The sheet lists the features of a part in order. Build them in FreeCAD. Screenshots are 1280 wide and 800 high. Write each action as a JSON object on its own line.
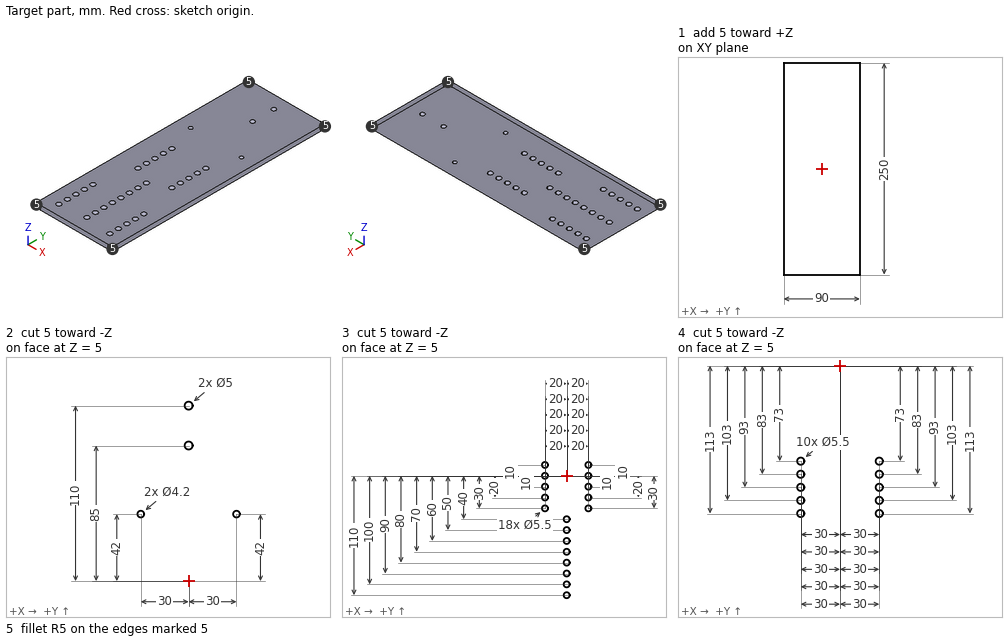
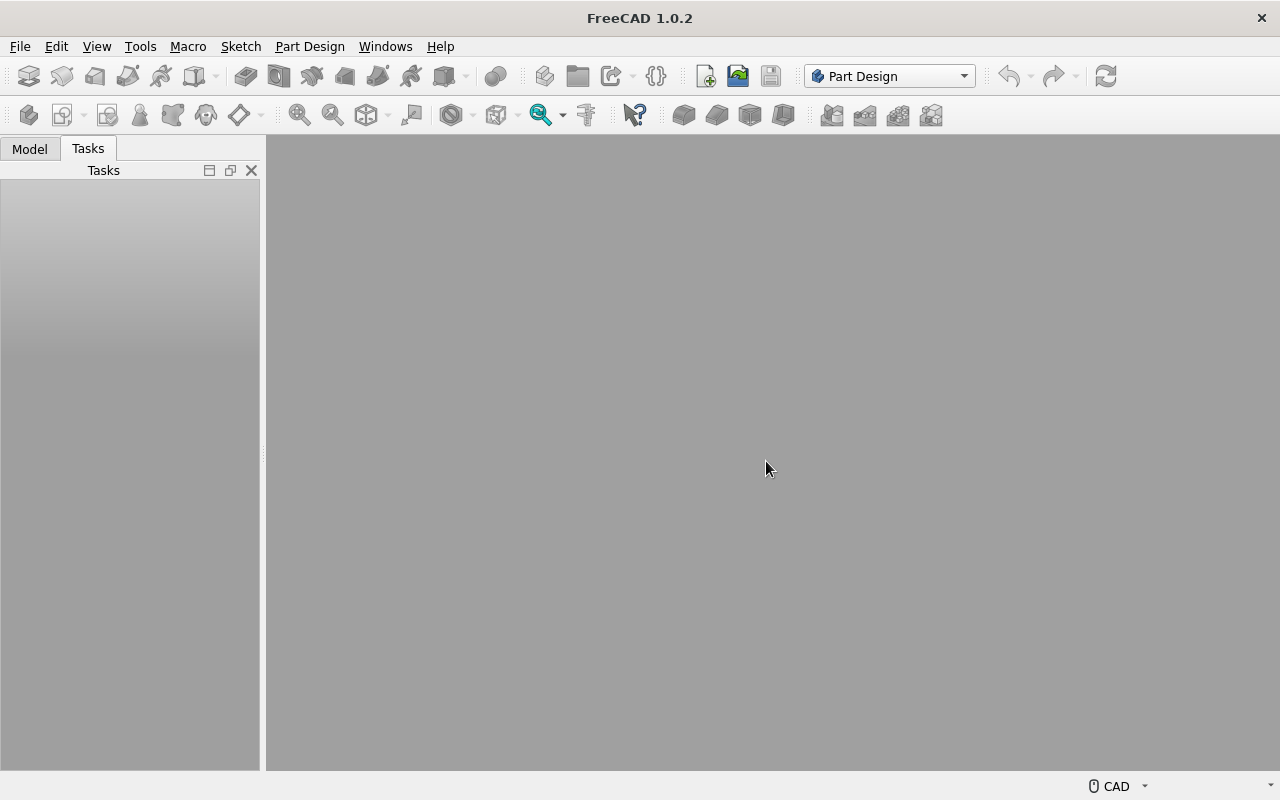
{"action": "key", "text": "ctrl+n"}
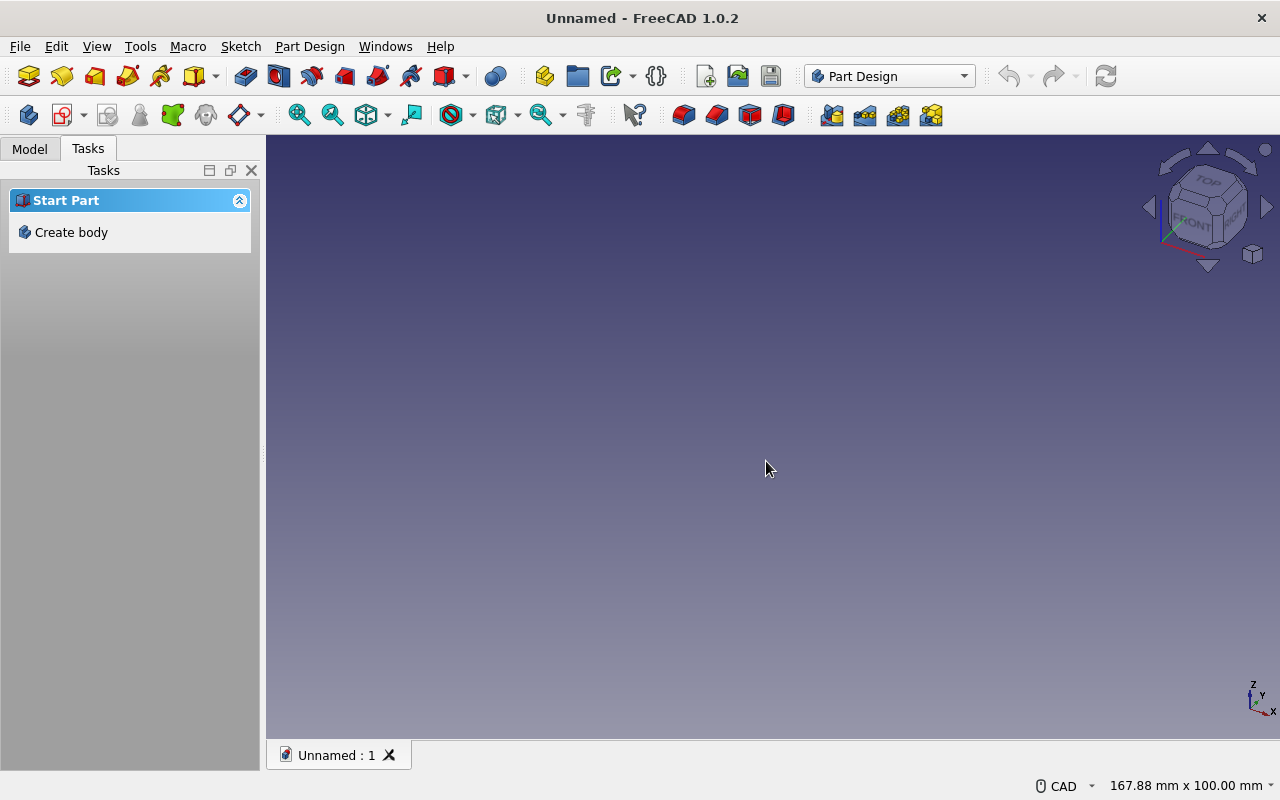
{"action": "left_click", "coordinate": [62, 116]}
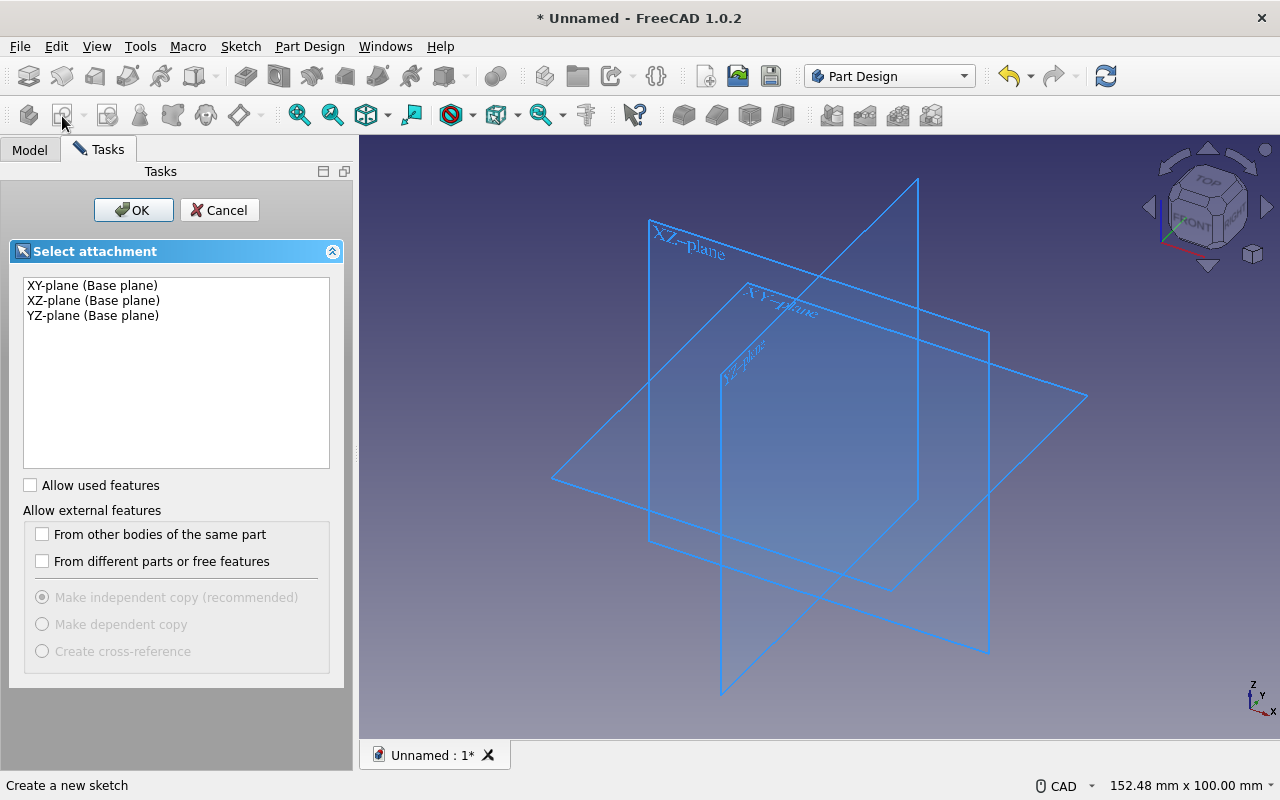
{"action": "left_click", "coordinate": [84, 286]}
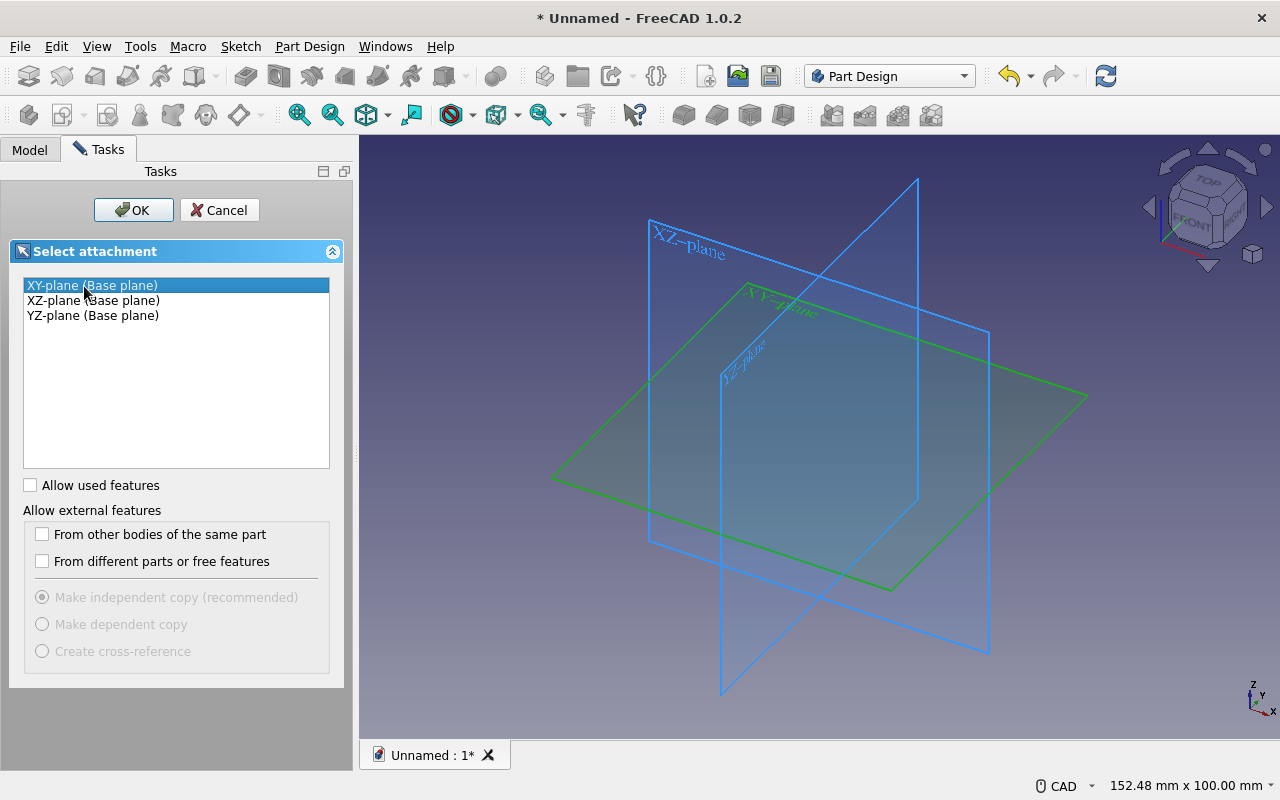
{"action": "left_click", "coordinate": [134, 210]}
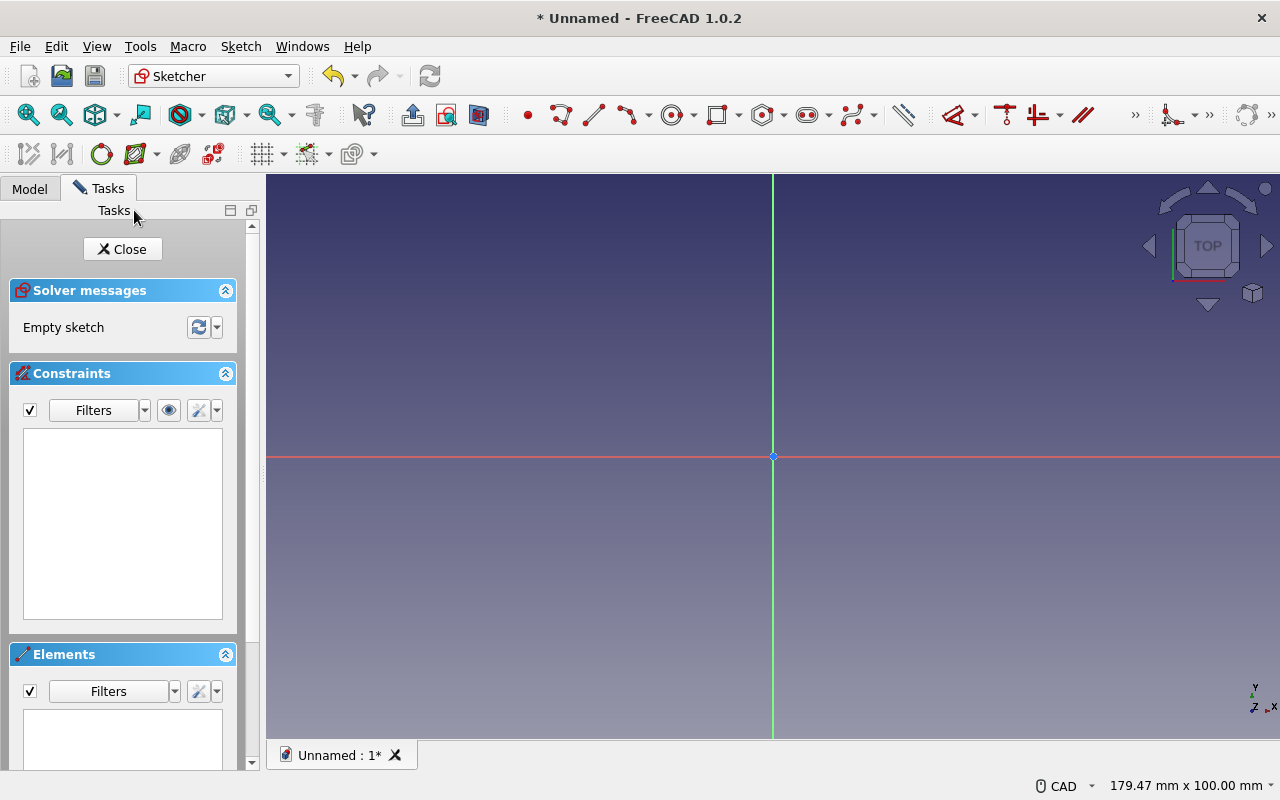
{"action": "scroll", "coordinate": [682, 456], "scroll_direction": "down", "scroll_amount": 7}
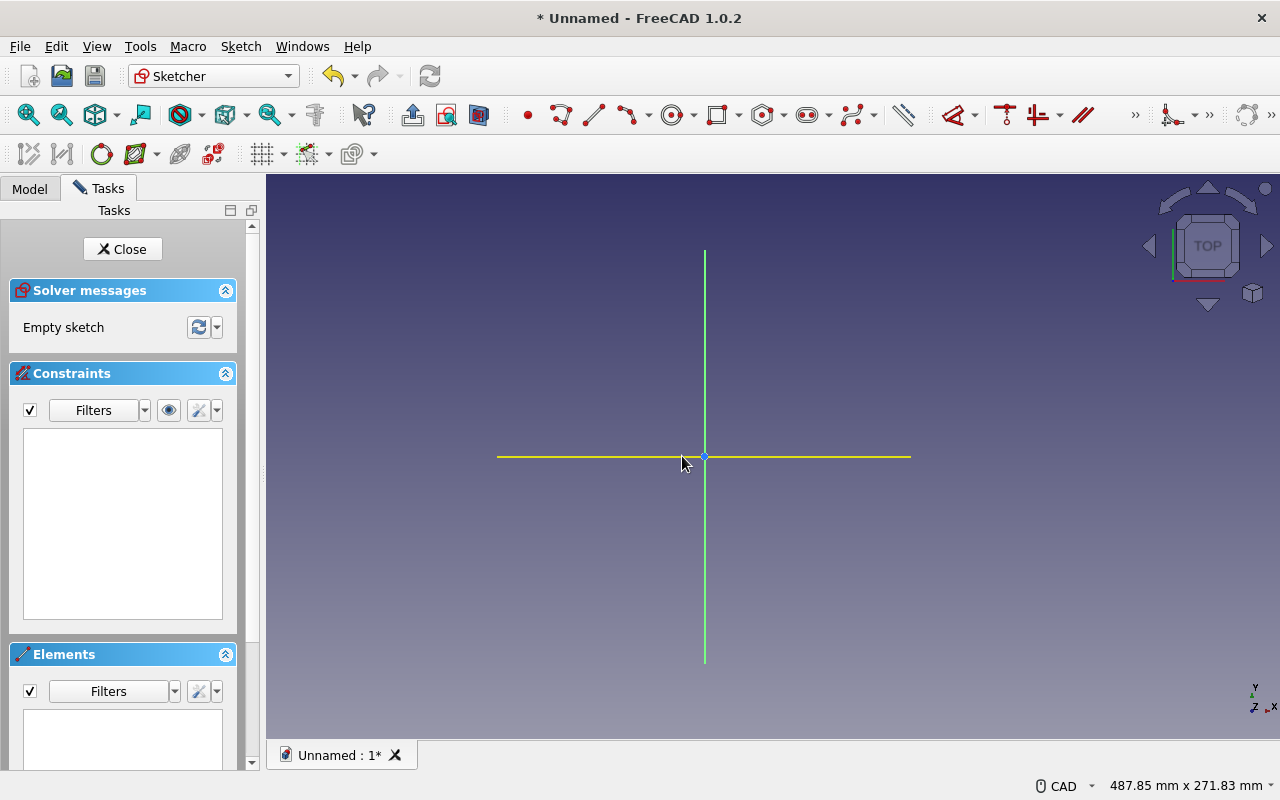
{"action": "left_click", "coordinate": [738, 116]}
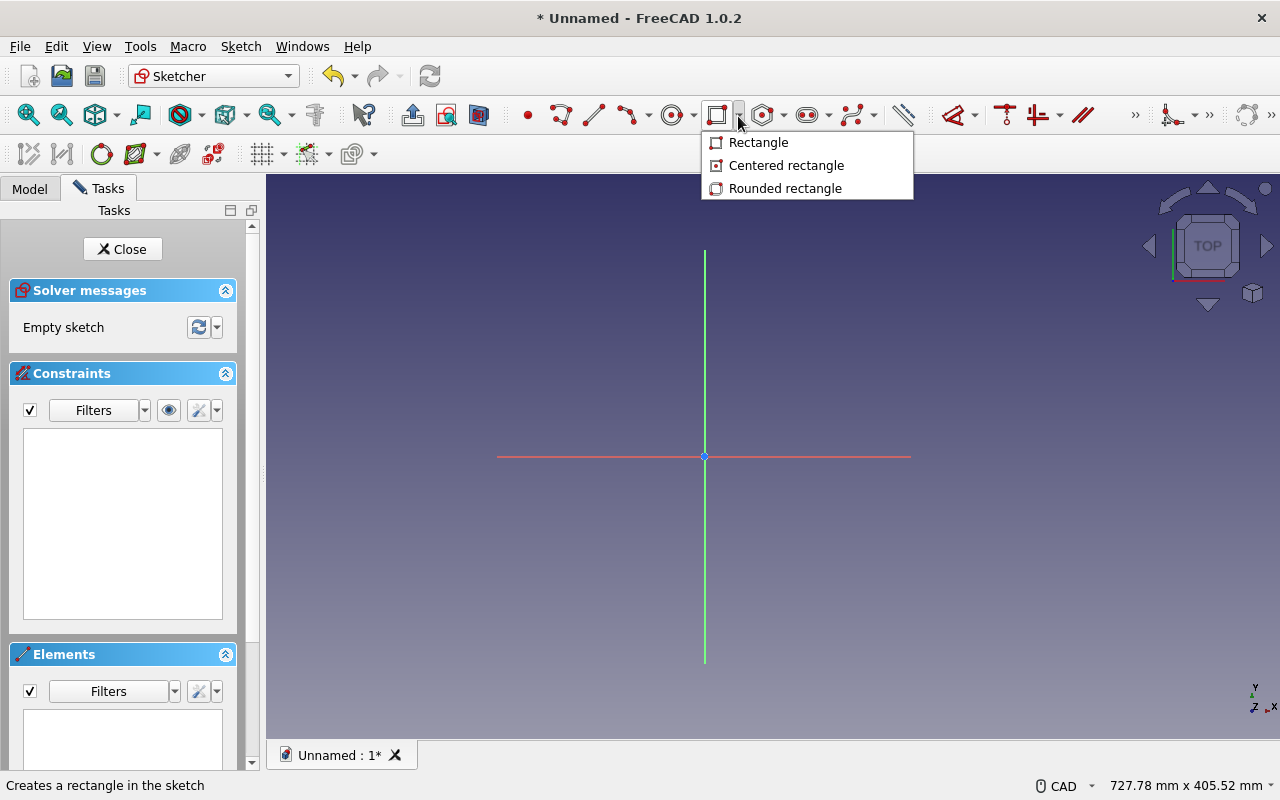
{"action": "left_click", "coordinate": [808, 166]}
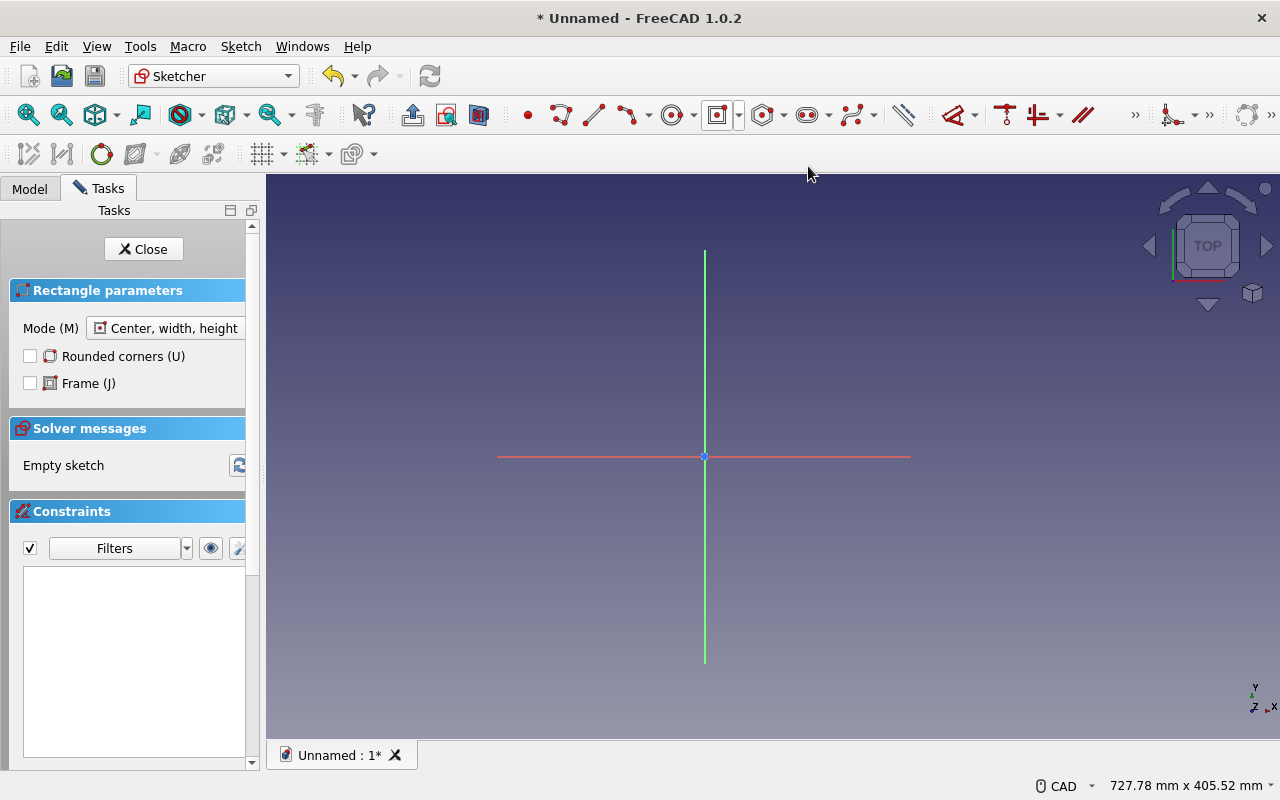
{"action": "left_click", "coordinate": [705, 456]}
{"action": "mouse_move", "coordinate": [767, 282]}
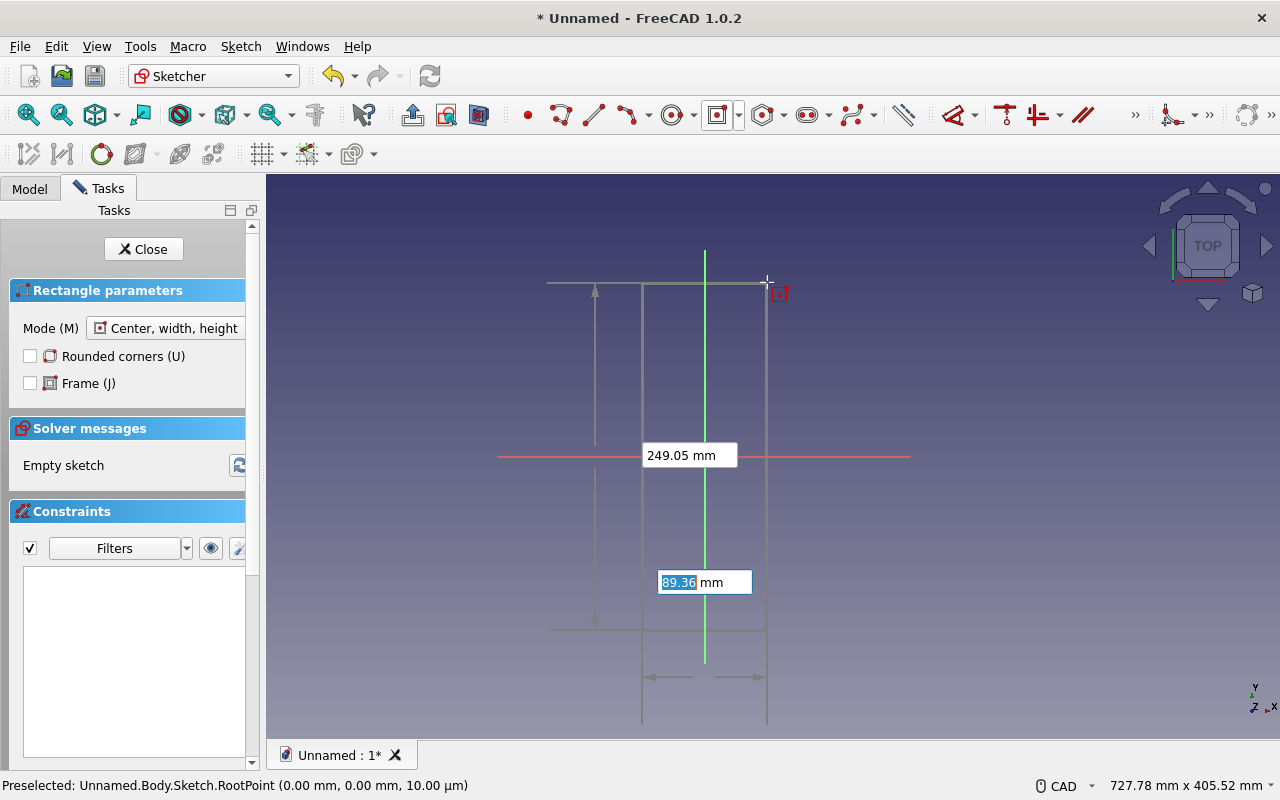
{"action": "type", "text": "90"}
{"action": "key", "text": "Tab"}
{"action": "type", "text": "250"}
{"action": "key", "text": "Return"}
{"action": "key", "text": "Escape"}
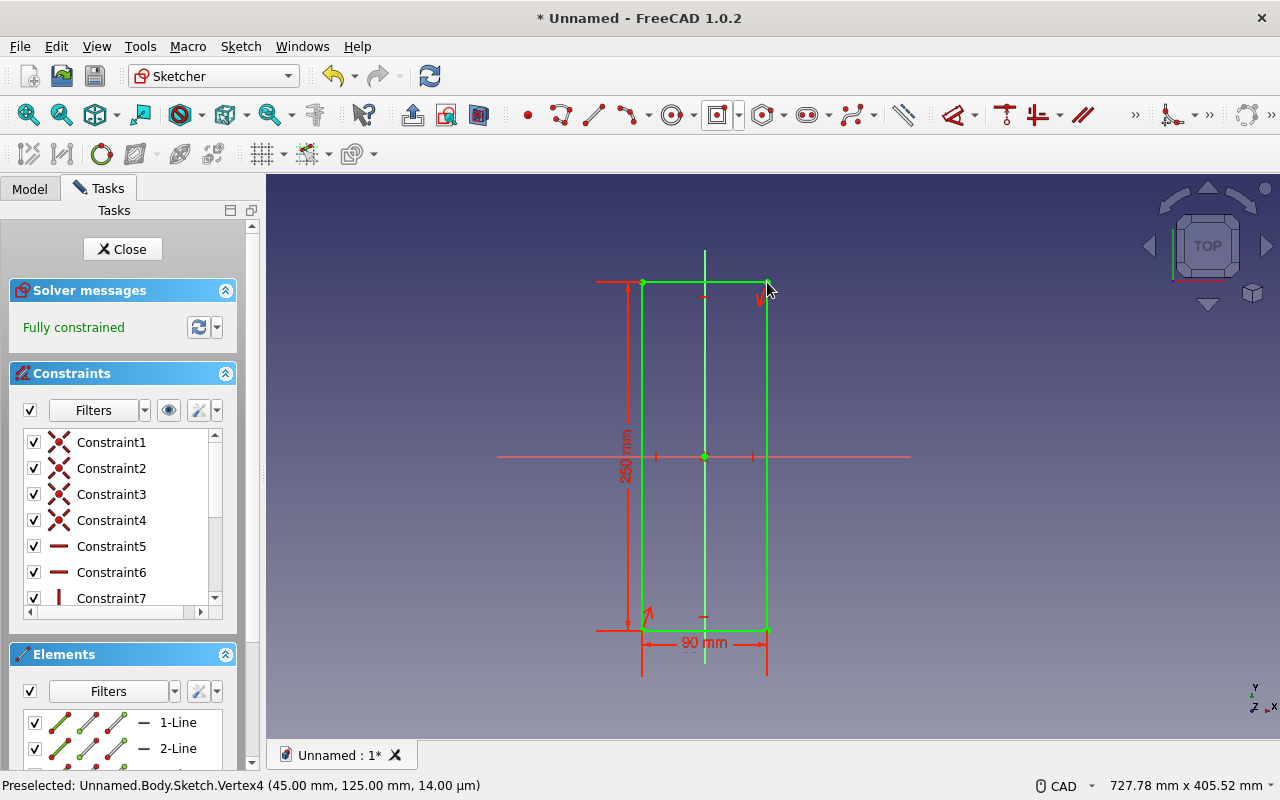
{"action": "left_click", "coordinate": [123, 249]}